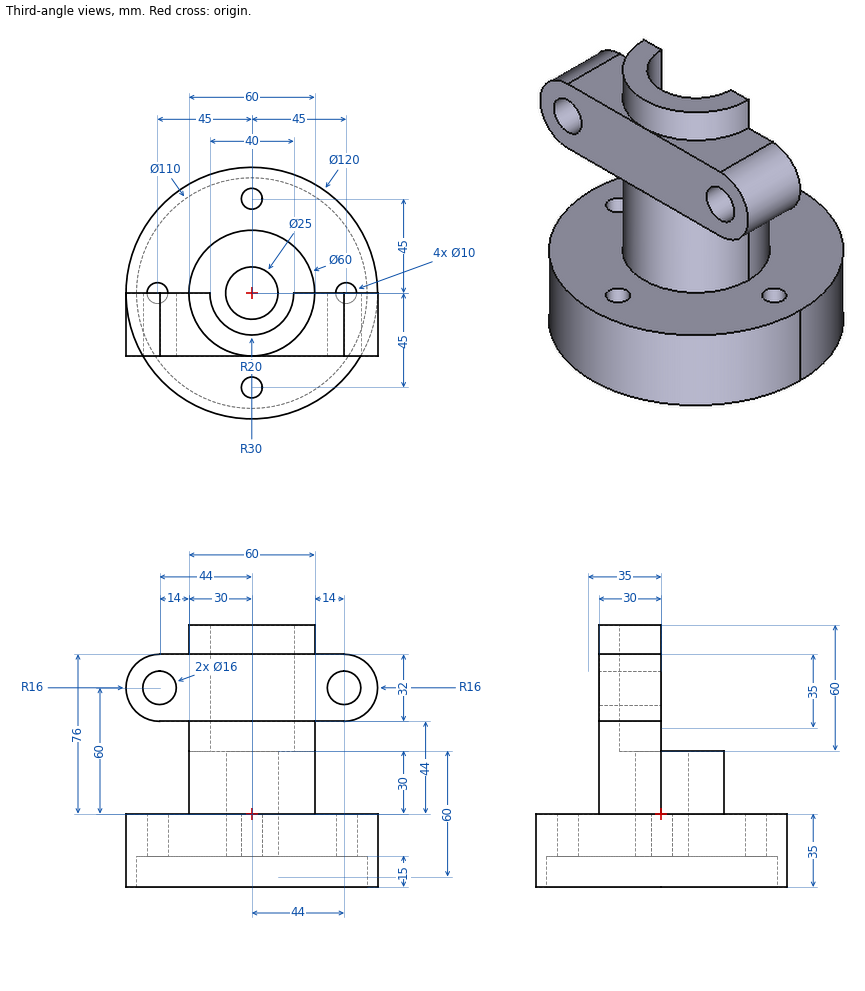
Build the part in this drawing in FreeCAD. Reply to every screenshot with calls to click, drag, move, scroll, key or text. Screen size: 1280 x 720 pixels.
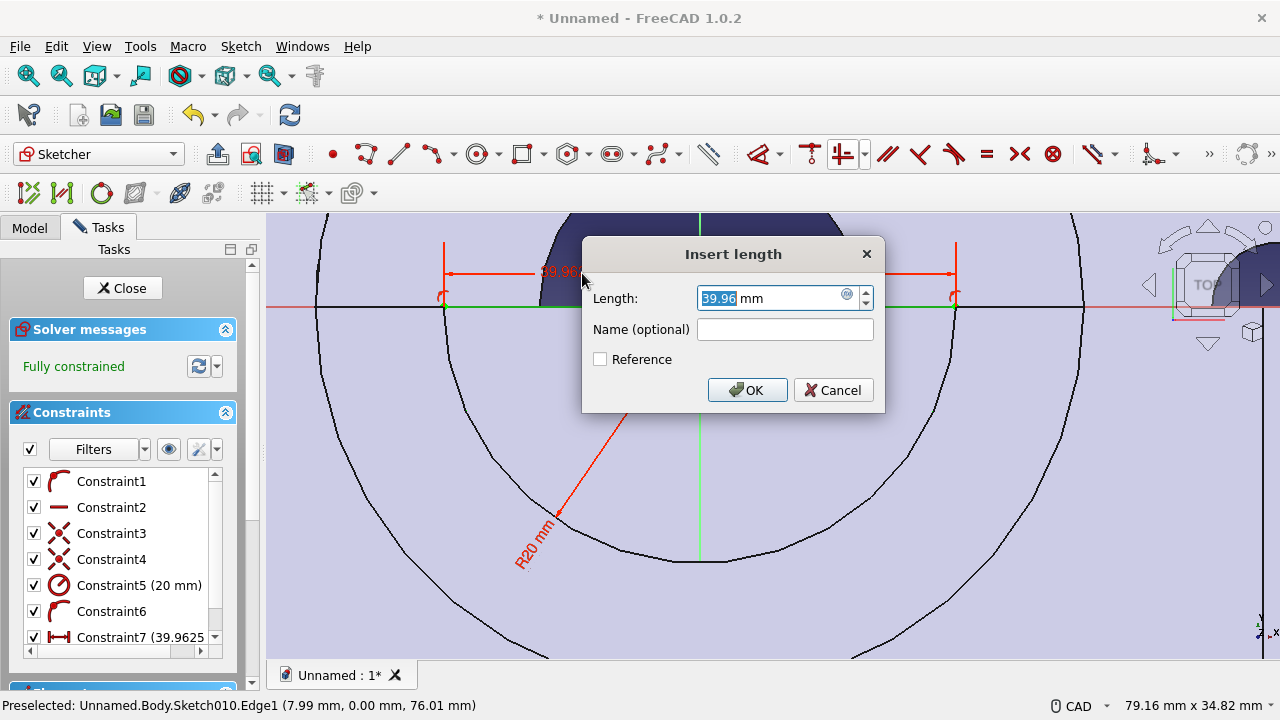
text(40)
key(Return)
key(Escape)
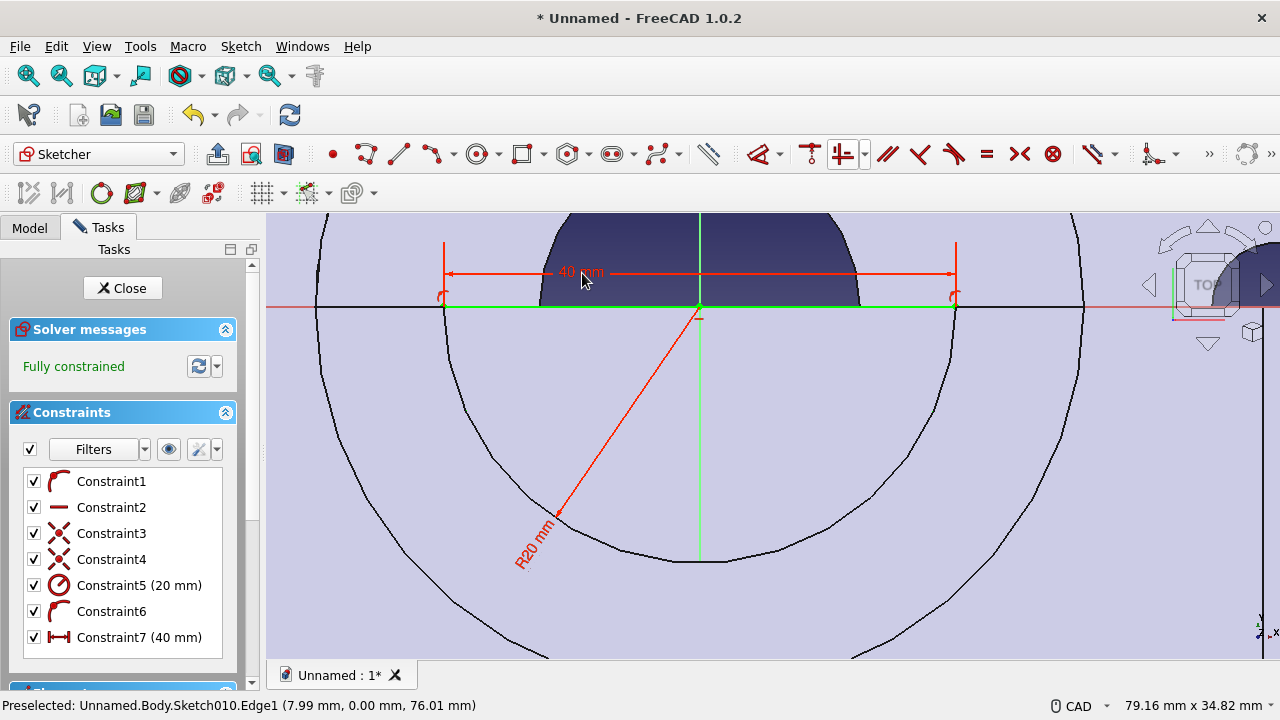
click(123, 288)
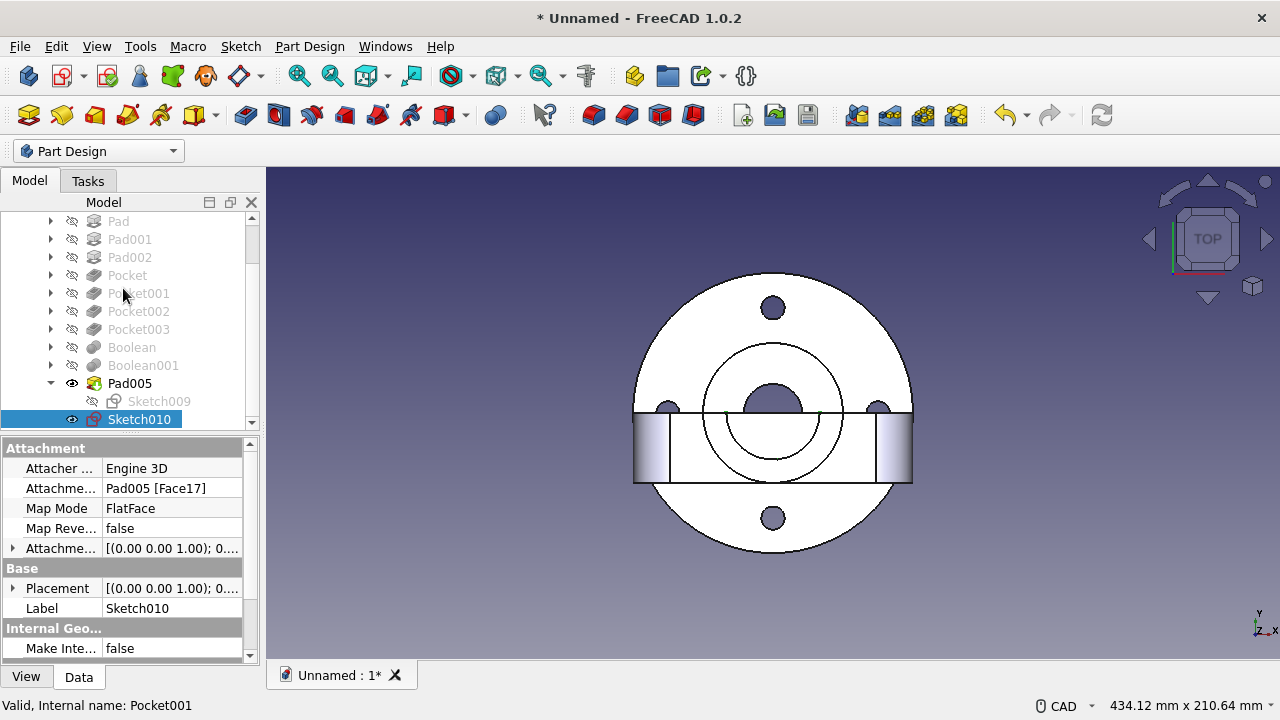
click(246, 116)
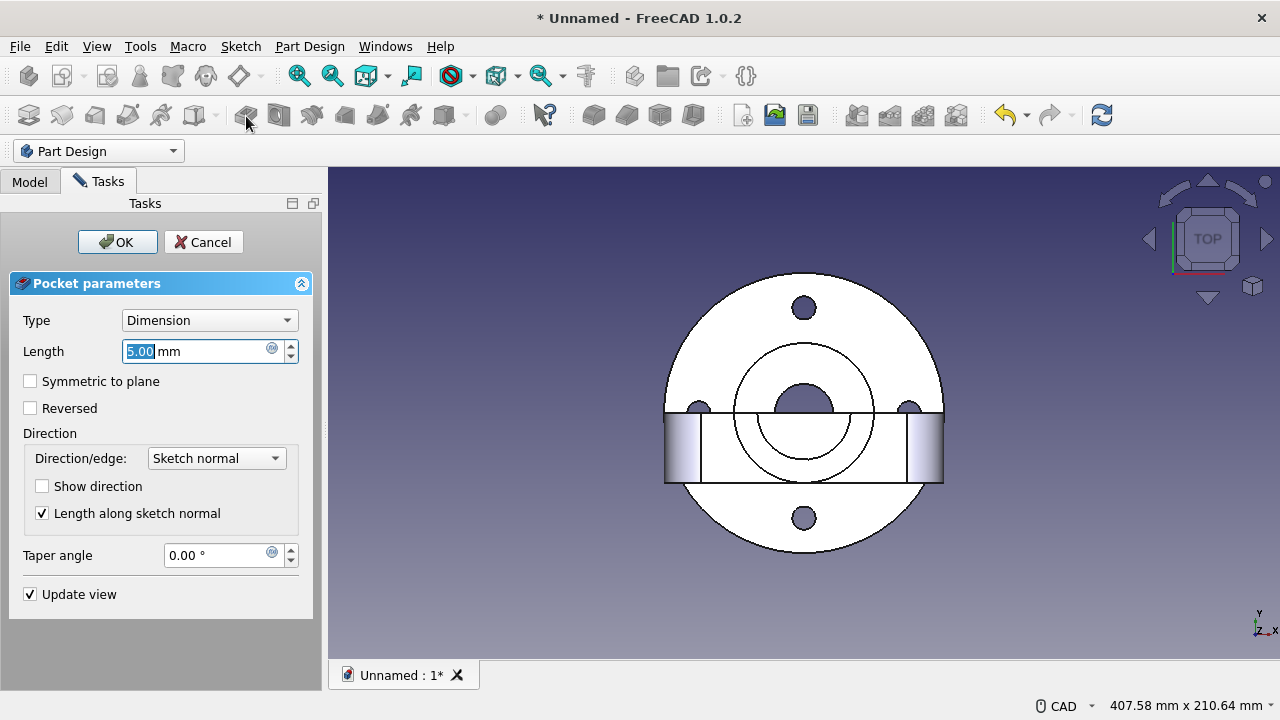
text(35)
key(Tab)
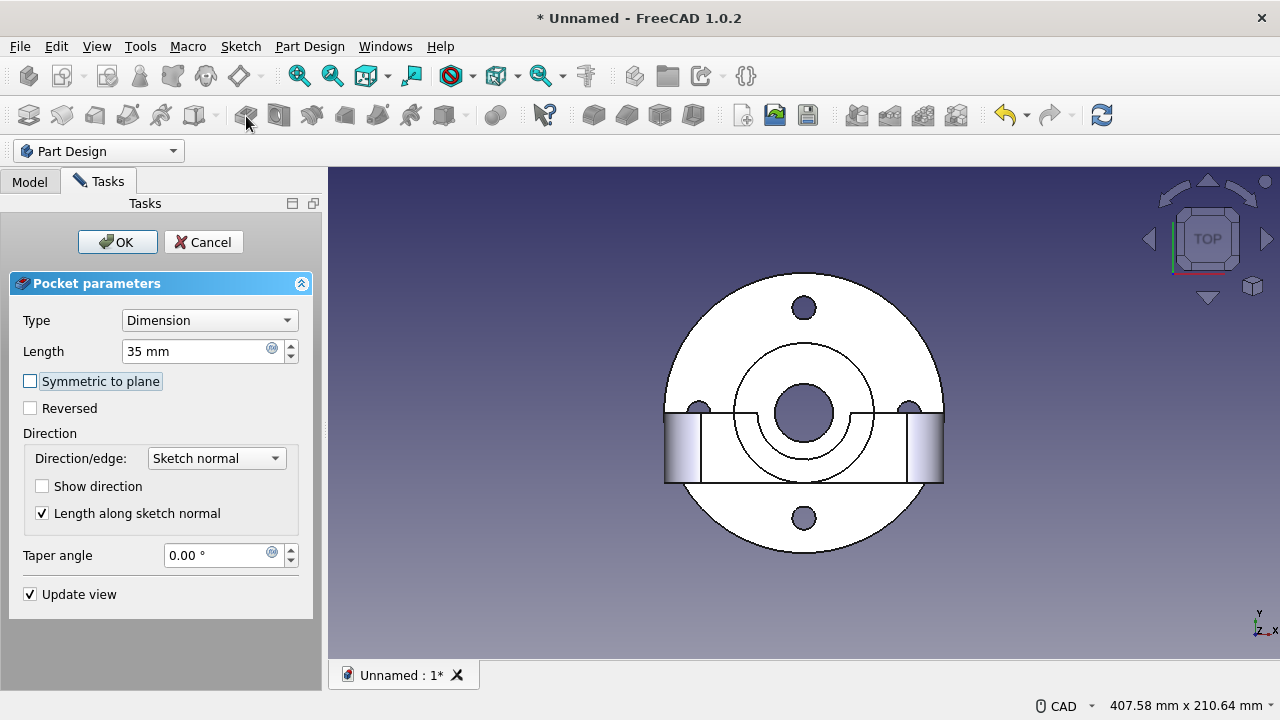
click(118, 242)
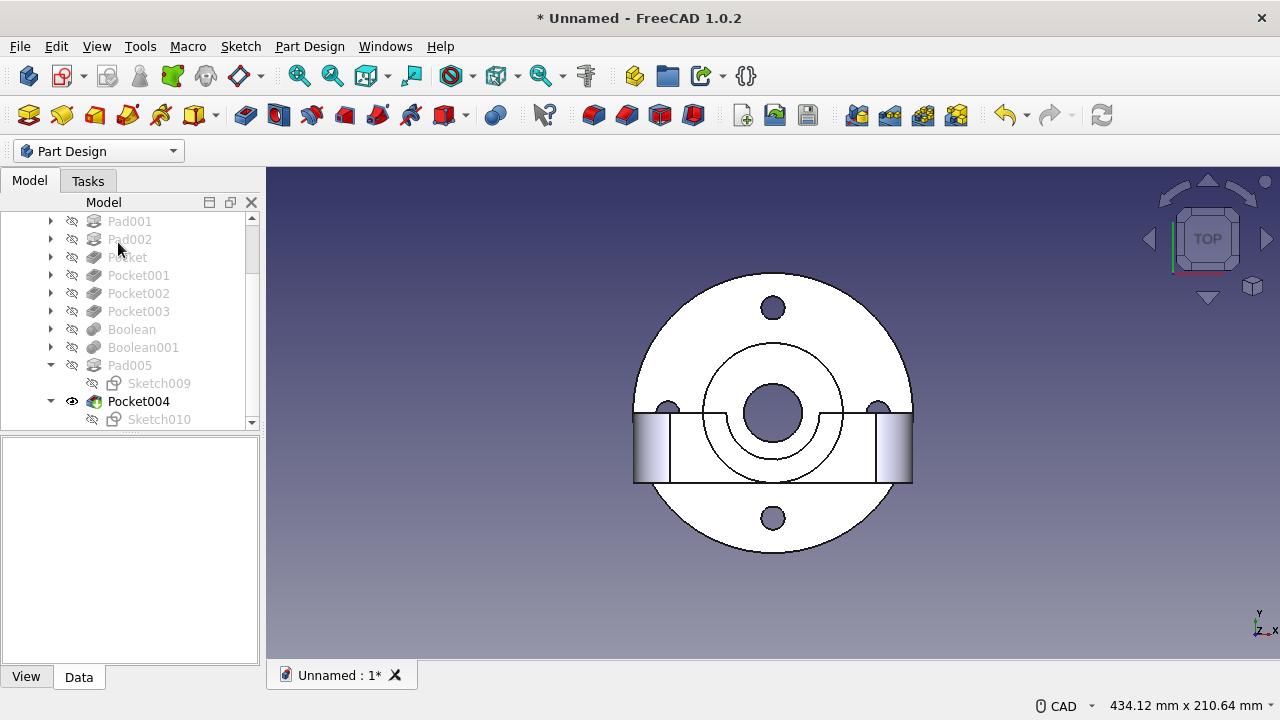
click(62, 76)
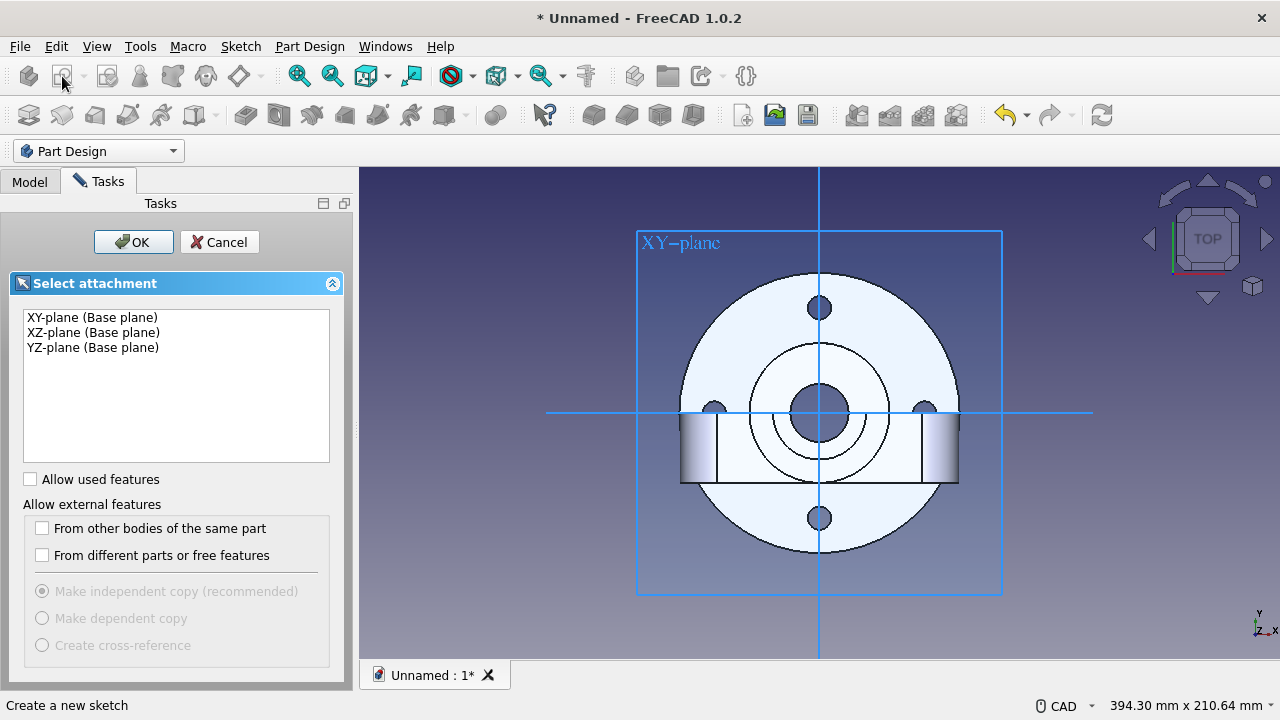
click(84, 332)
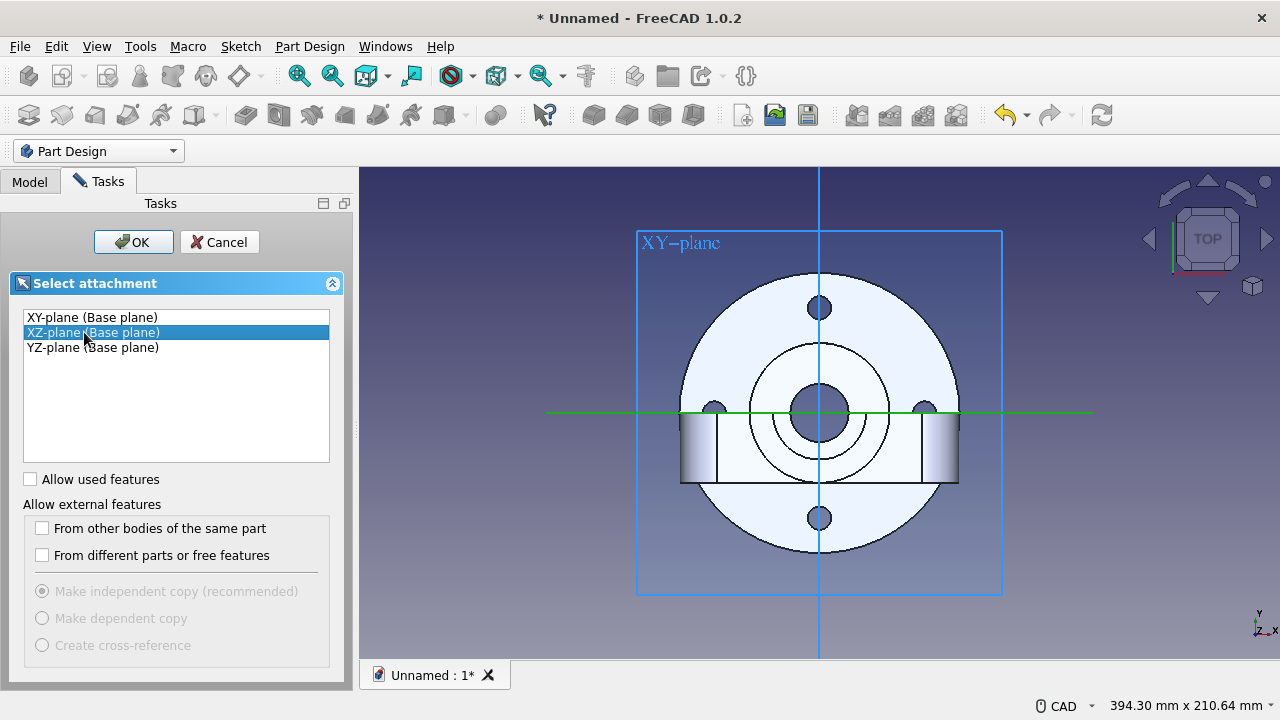
click(134, 242)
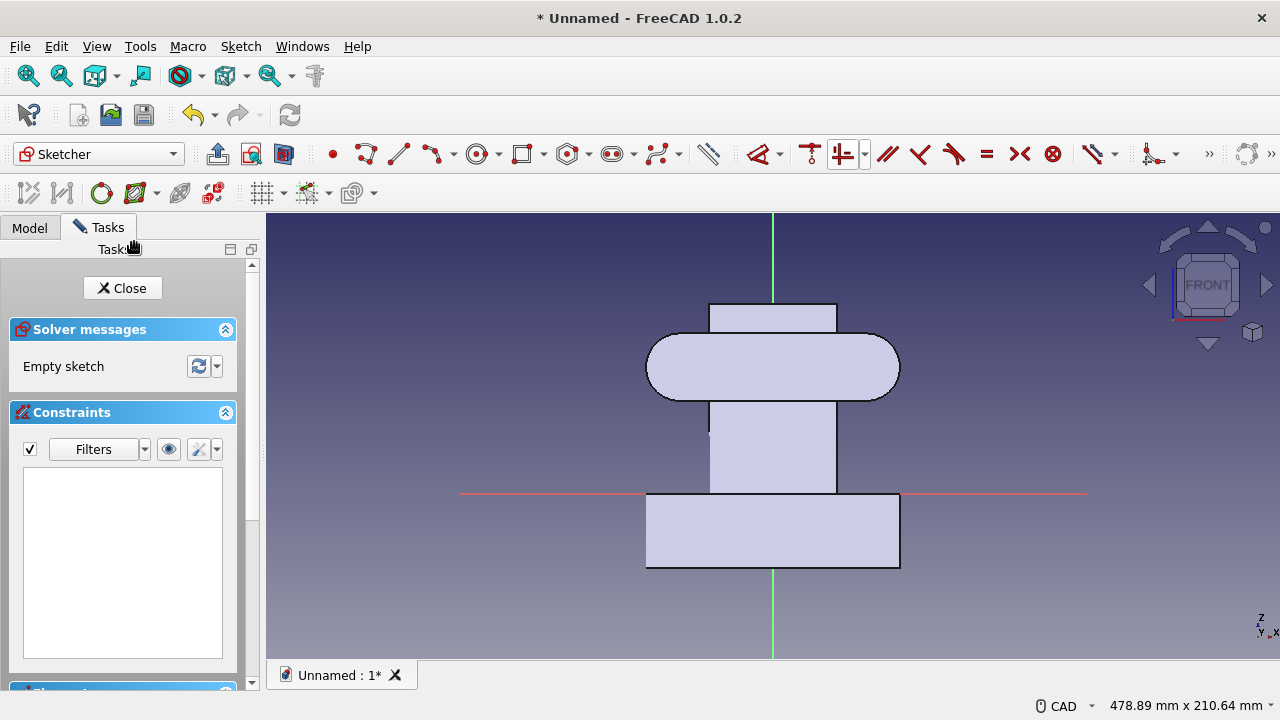
click(284, 154)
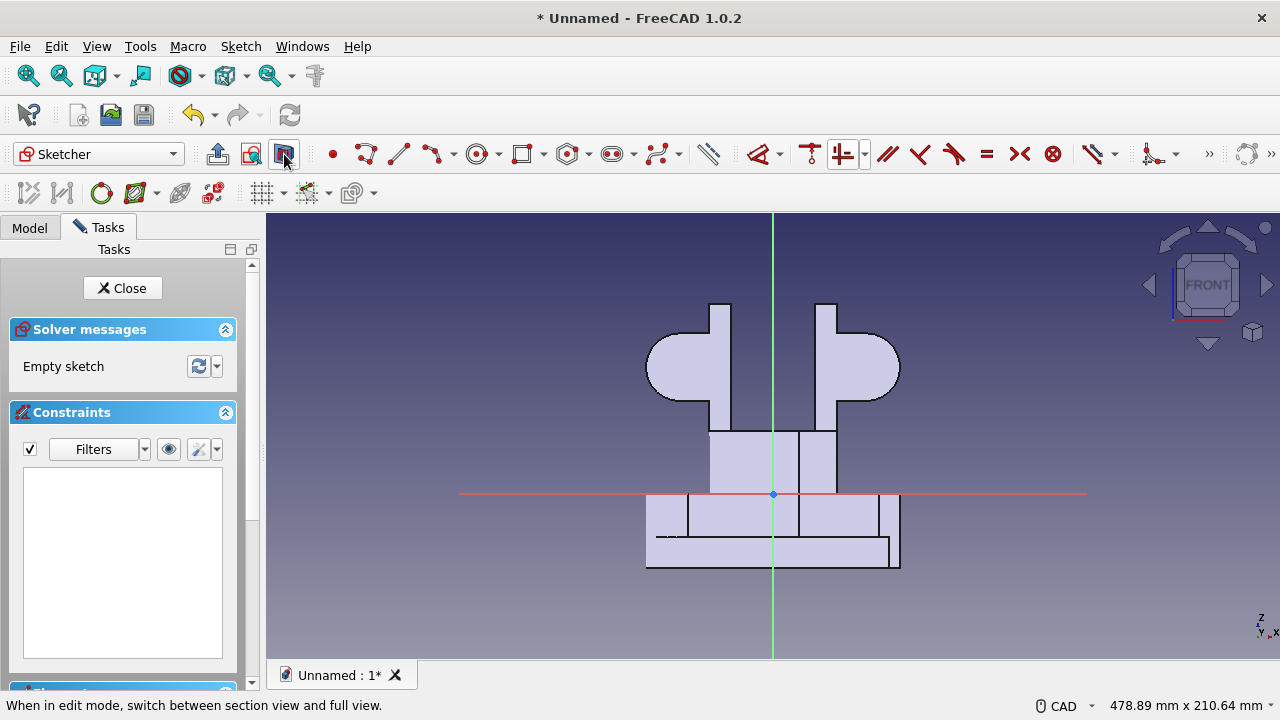
scroll(856, 405, up, 3)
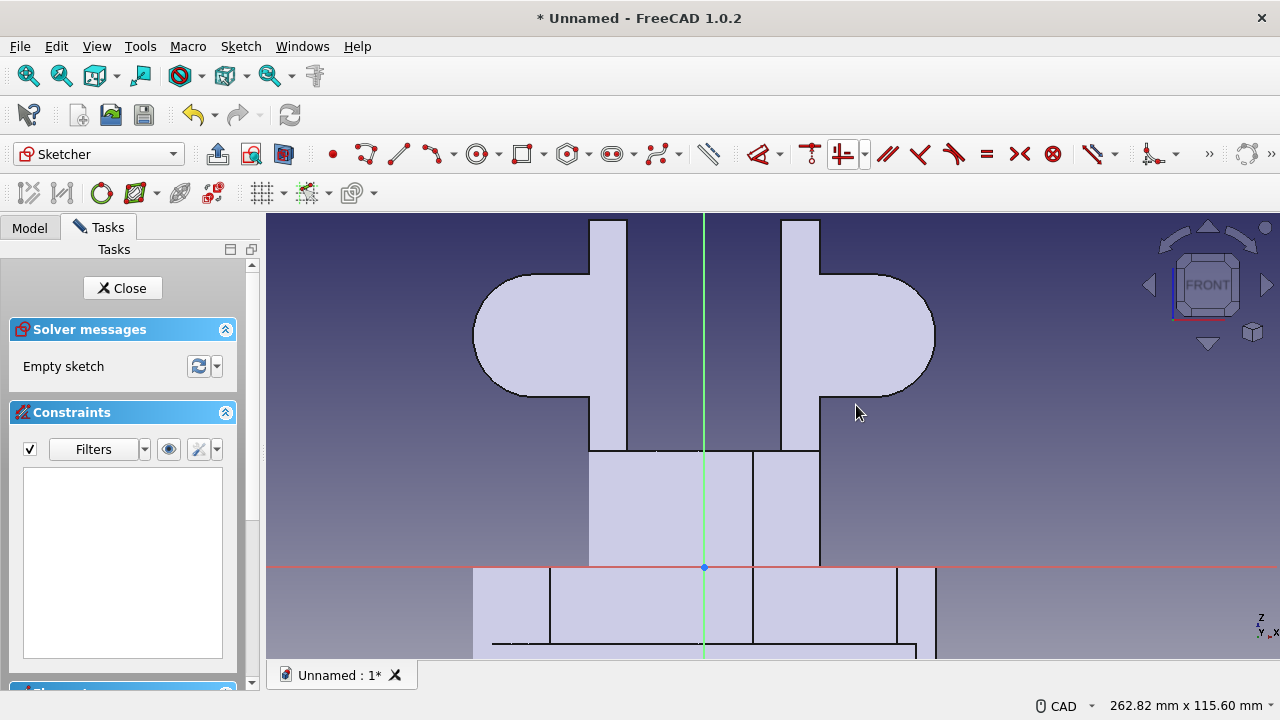
click(476, 154)